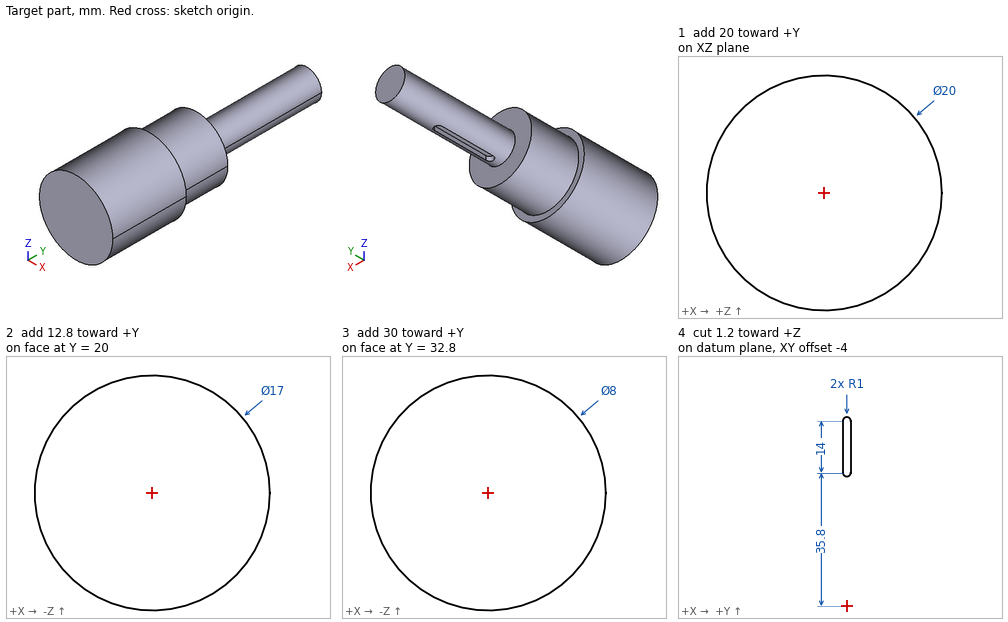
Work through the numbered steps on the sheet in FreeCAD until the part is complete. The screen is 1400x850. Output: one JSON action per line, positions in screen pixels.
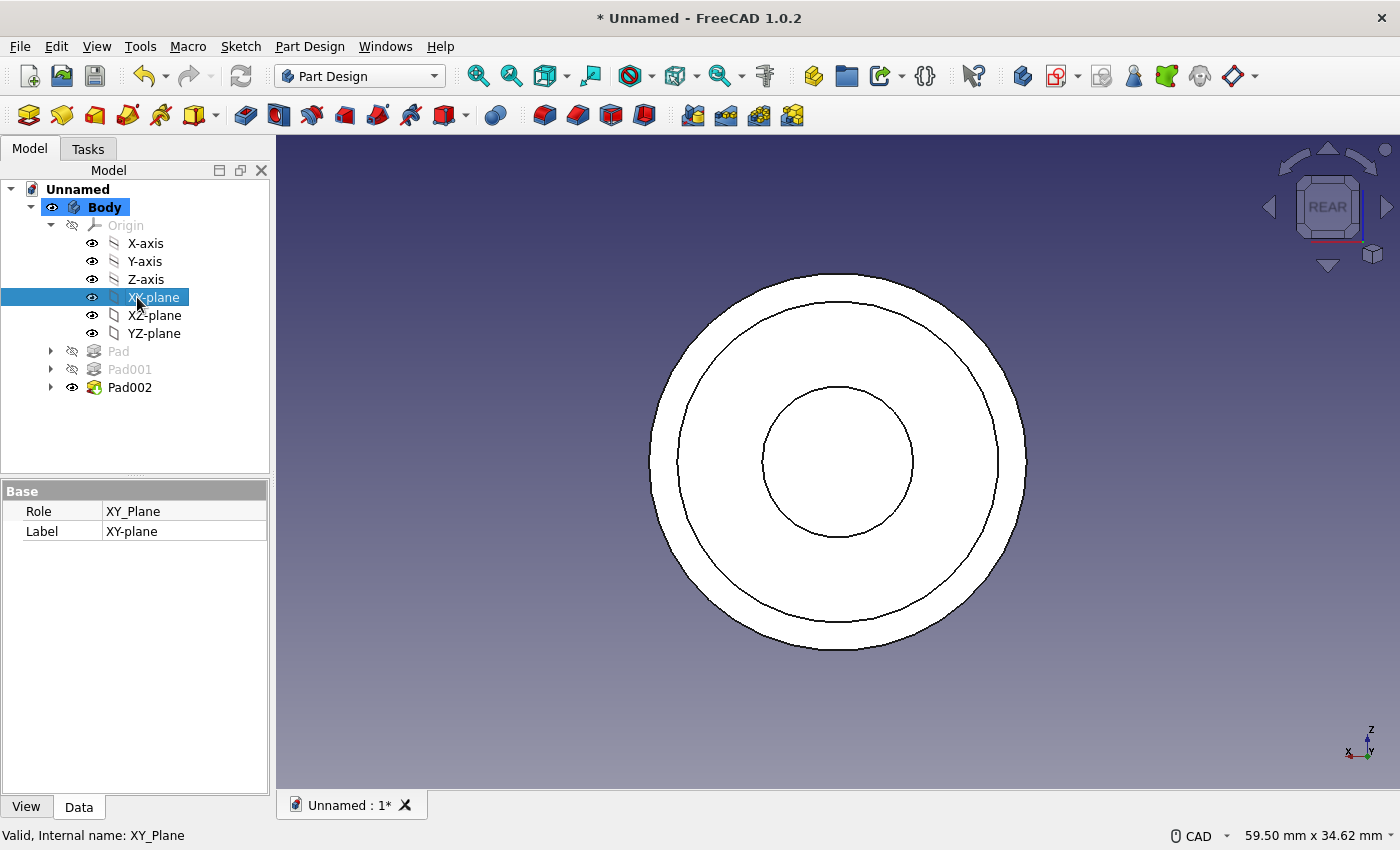
{"action": "left_click", "coordinate": [1232, 76]}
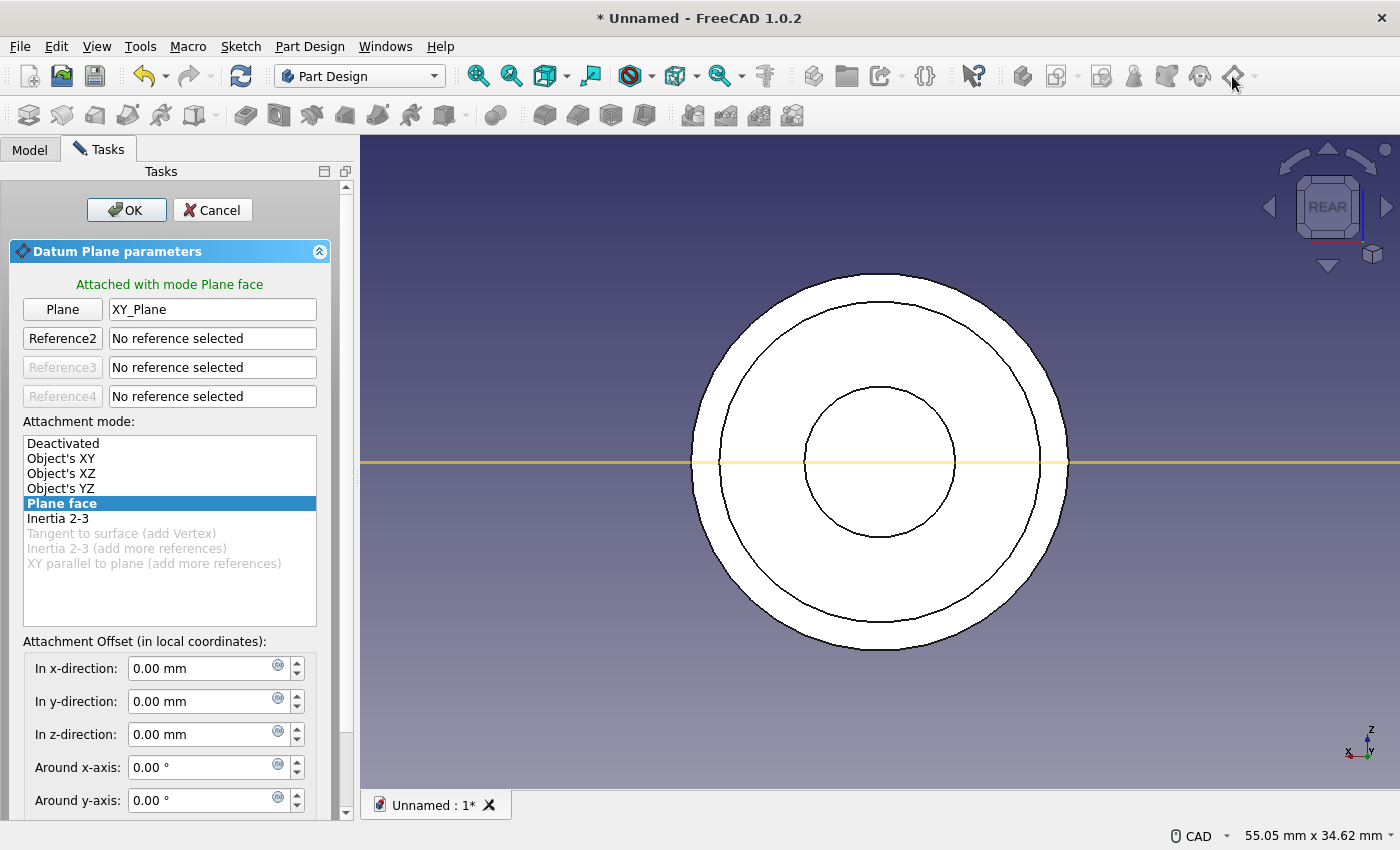
{"action": "triple_click", "coordinate": [210, 734]}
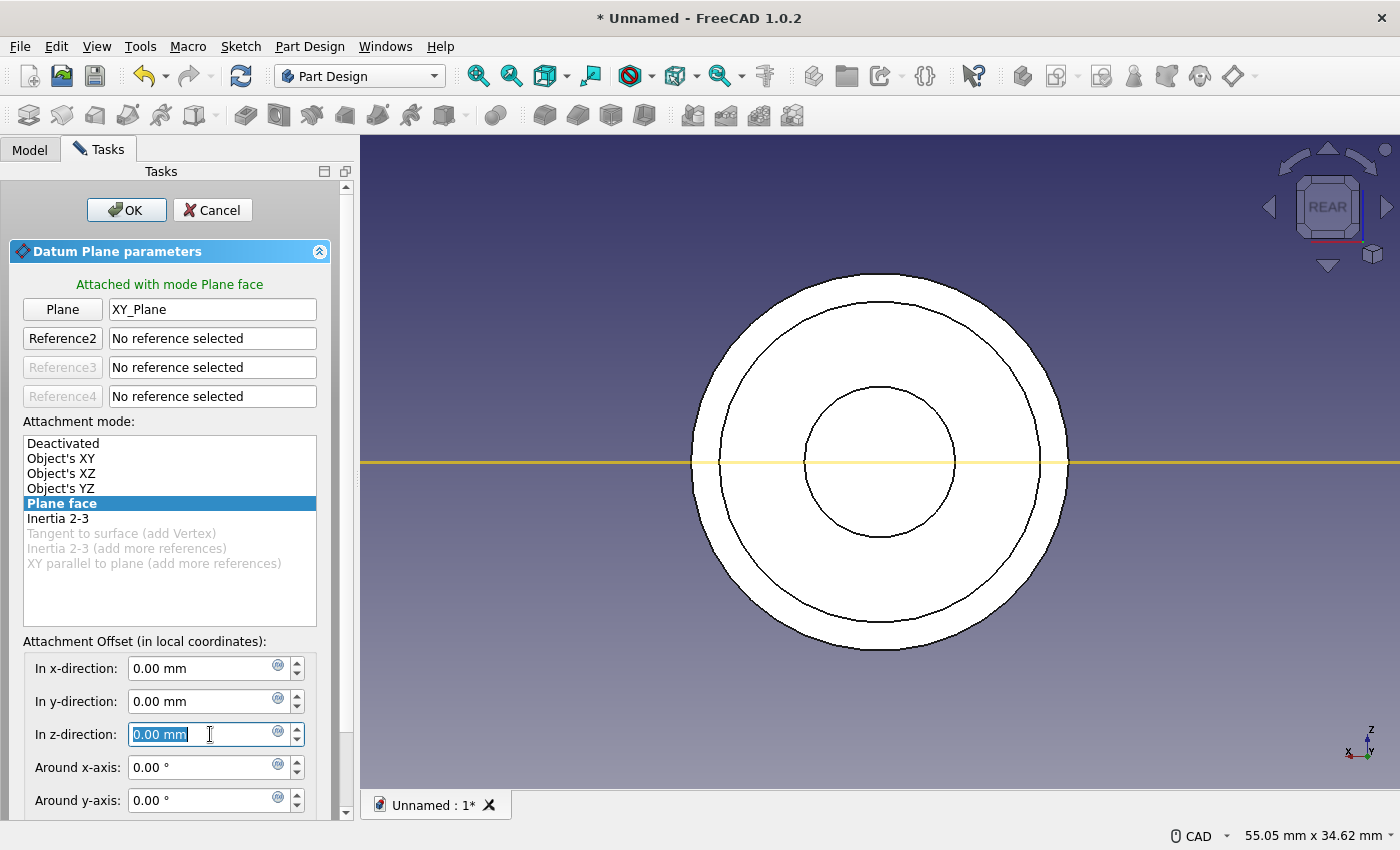
{"action": "type", "text": "-4"}
{"action": "key", "text": "Tab"}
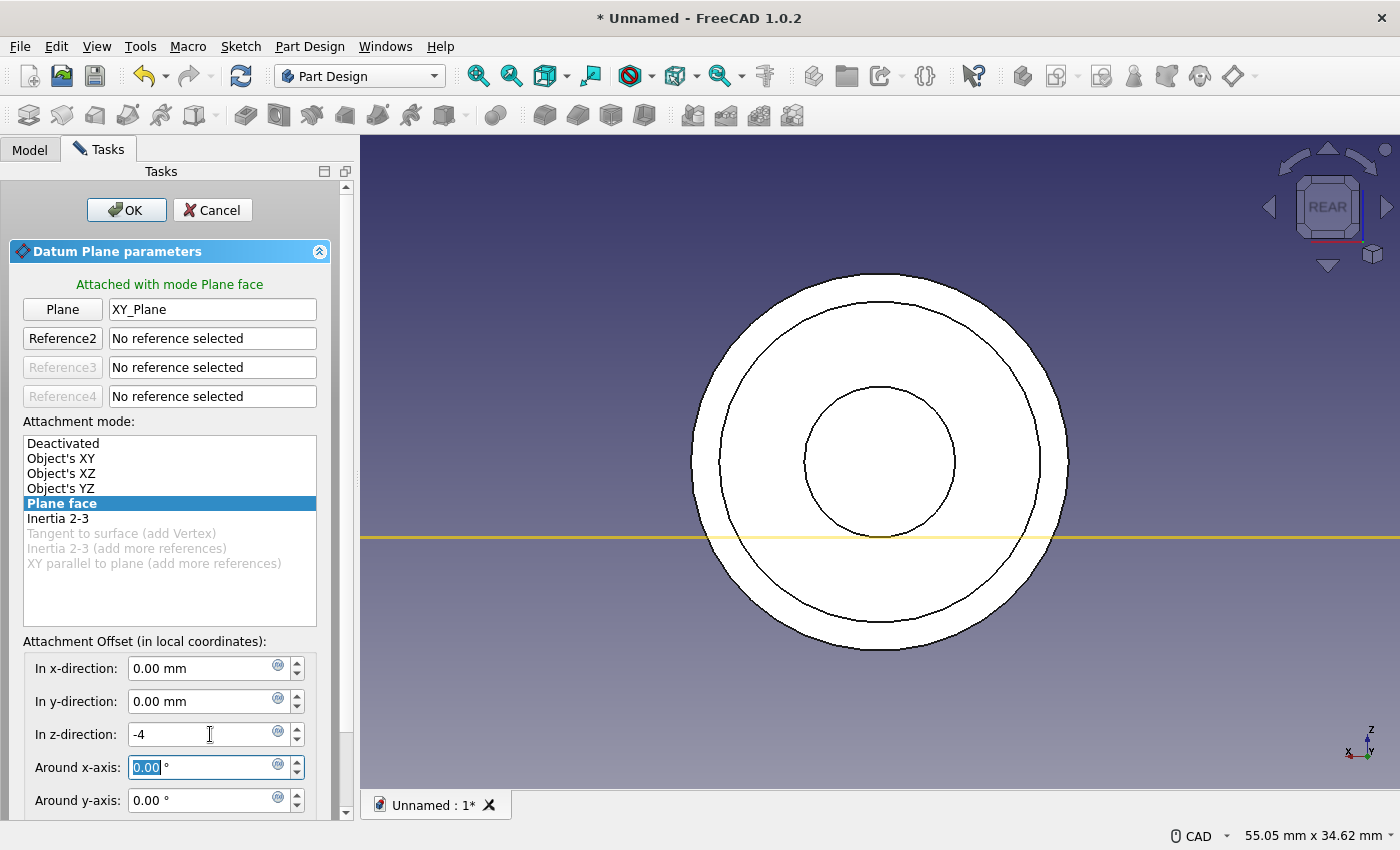
{"action": "left_click", "coordinate": [127, 210]}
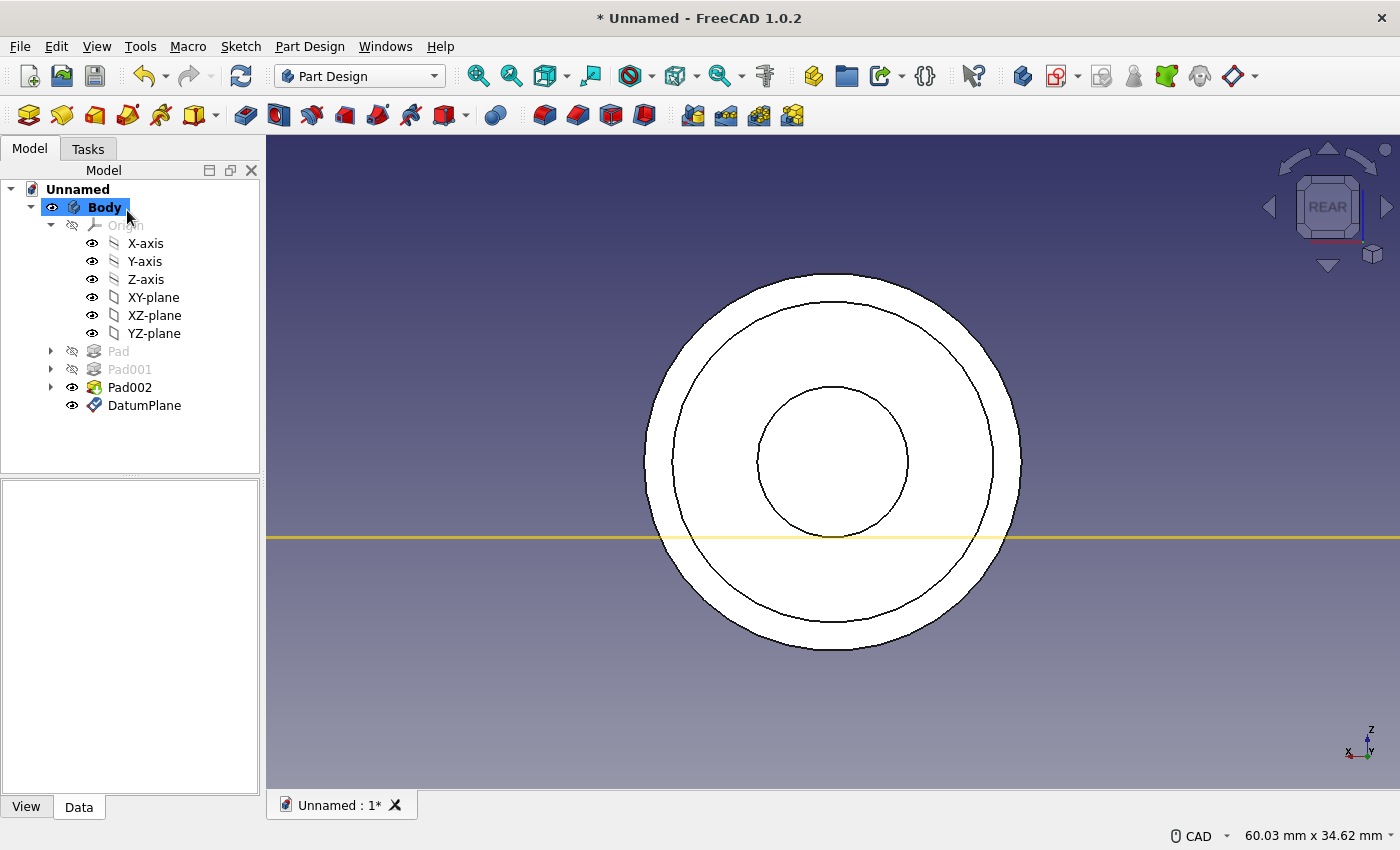
{"action": "left_click", "coordinate": [117, 405]}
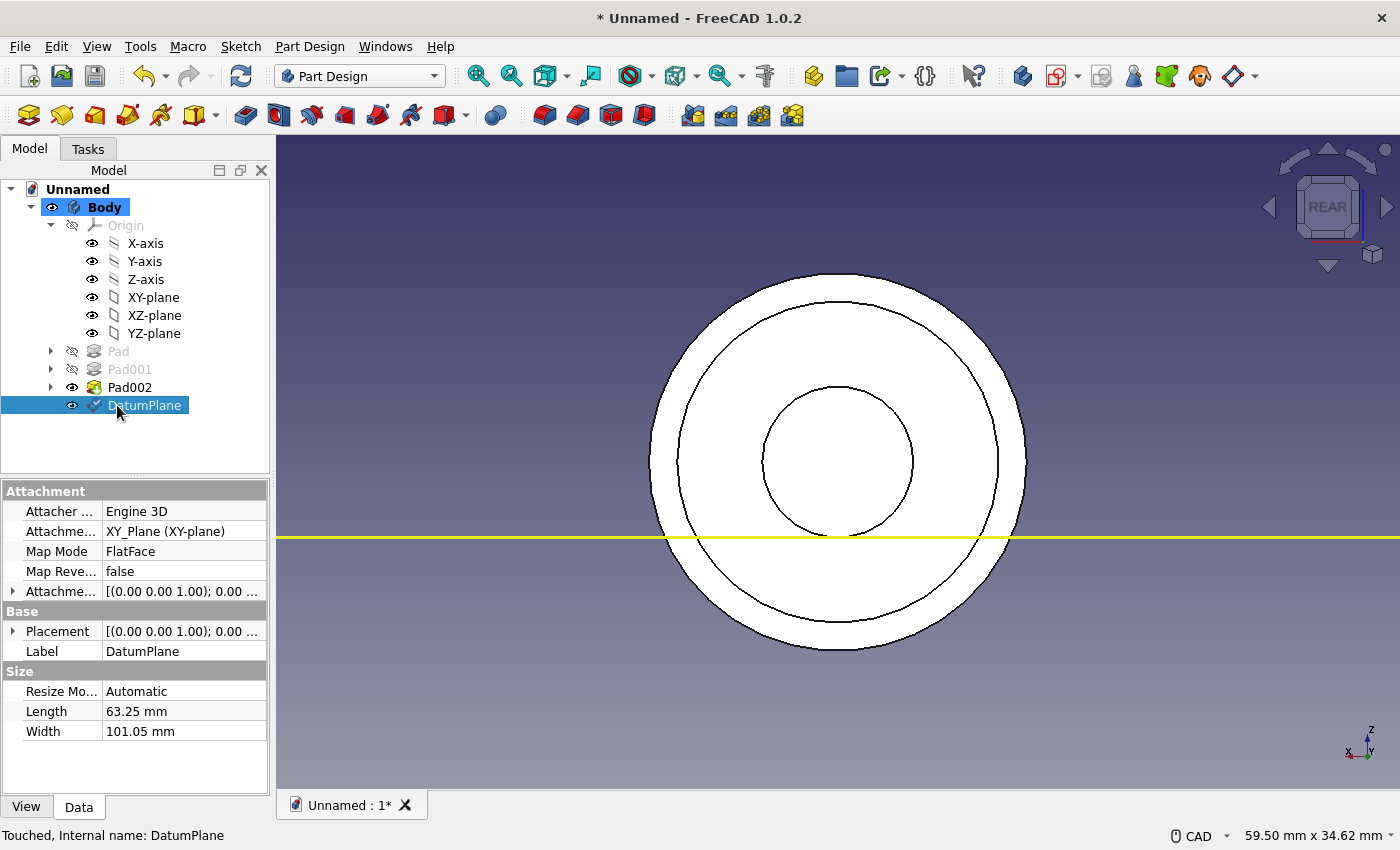
{"action": "left_click", "coordinate": [1056, 76]}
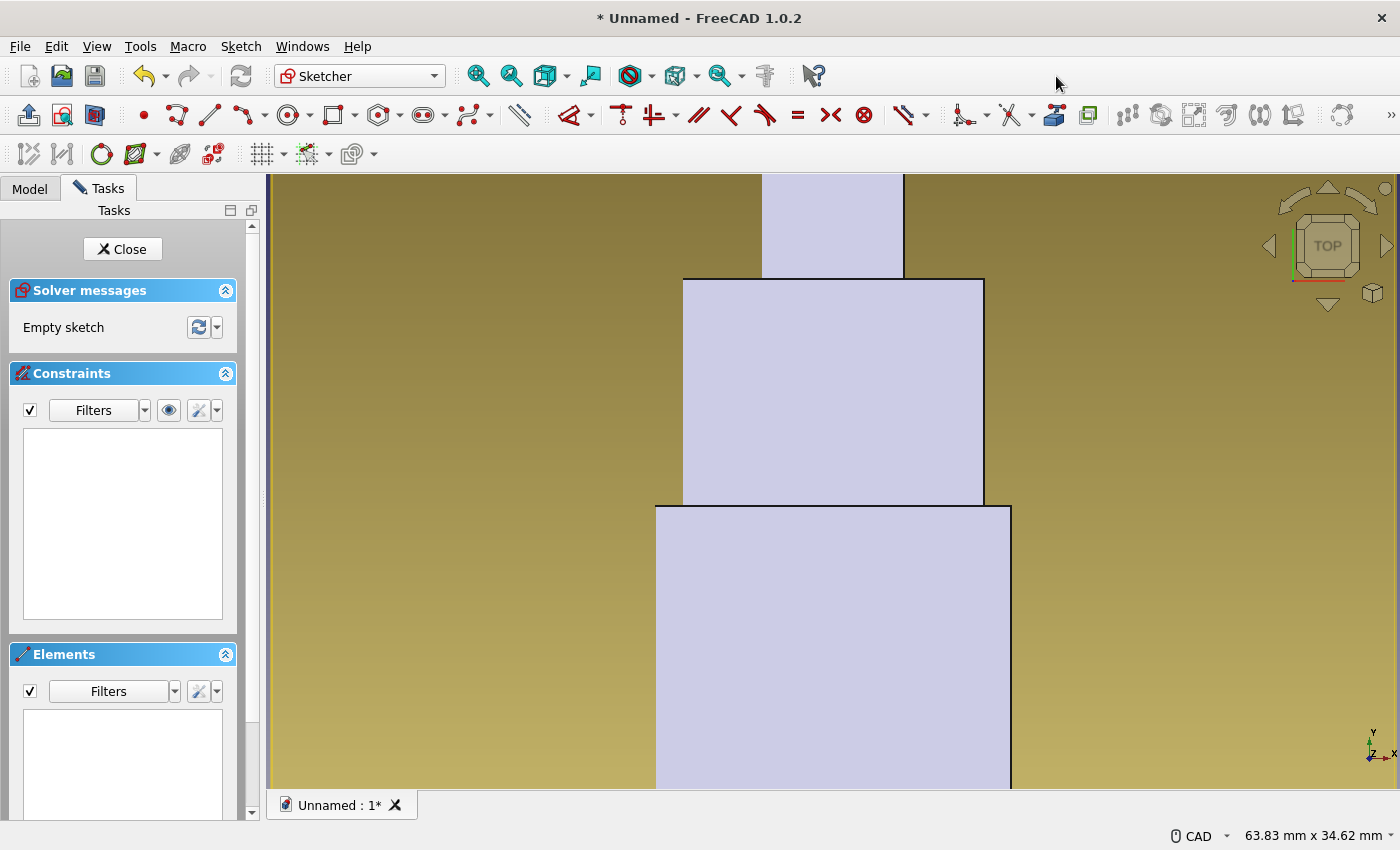
{"action": "left_click", "coordinate": [95, 116]}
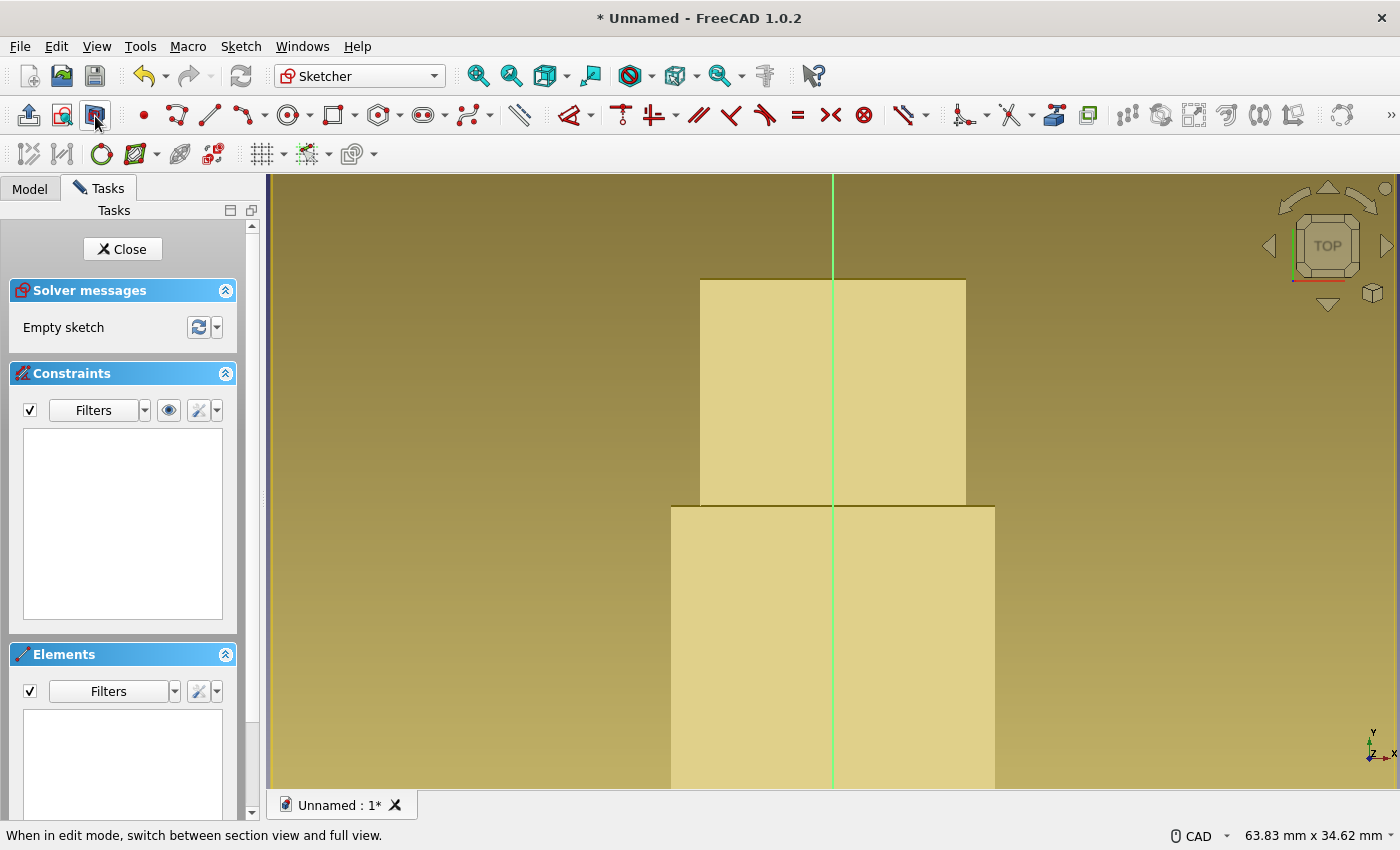
{"action": "scroll", "coordinate": [764, 482], "scroll_direction": "down", "scroll_amount": 5}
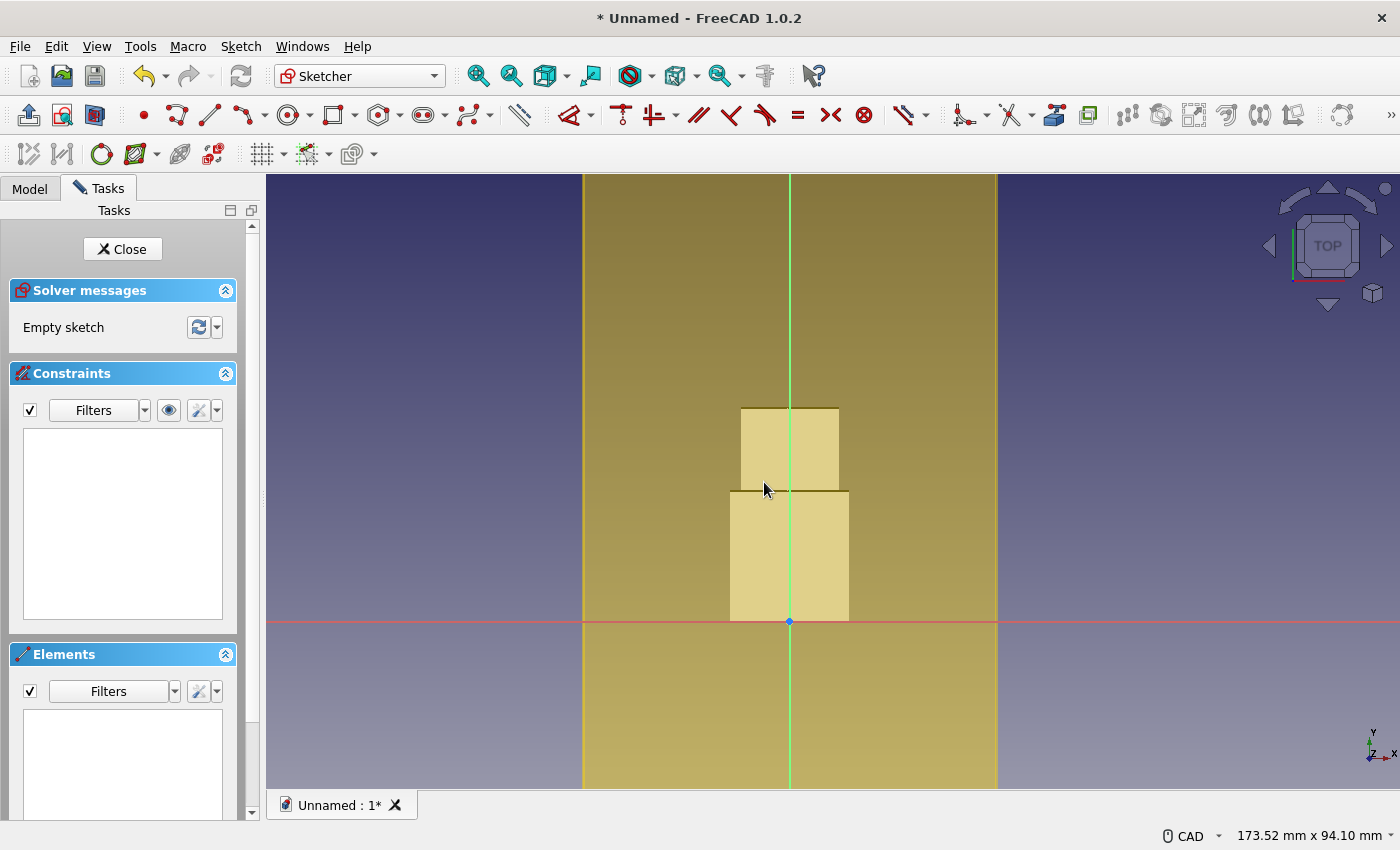
{"action": "scroll", "coordinate": [798, 297], "scroll_direction": "up", "scroll_amount": 7}